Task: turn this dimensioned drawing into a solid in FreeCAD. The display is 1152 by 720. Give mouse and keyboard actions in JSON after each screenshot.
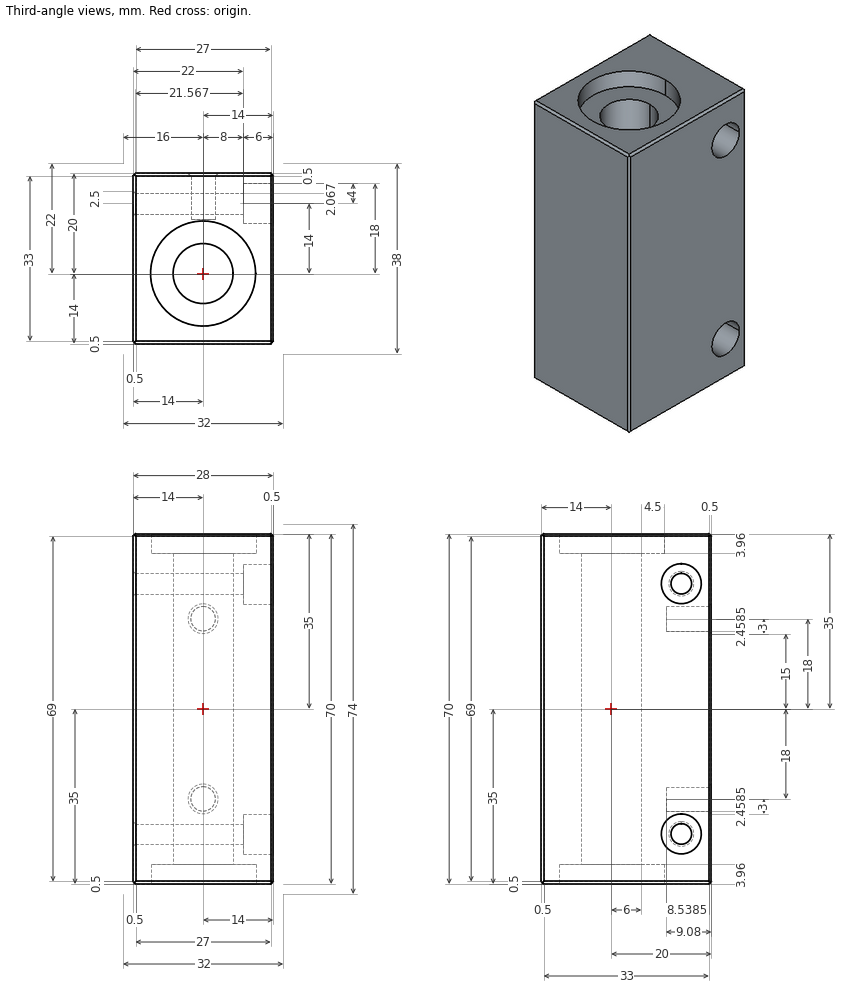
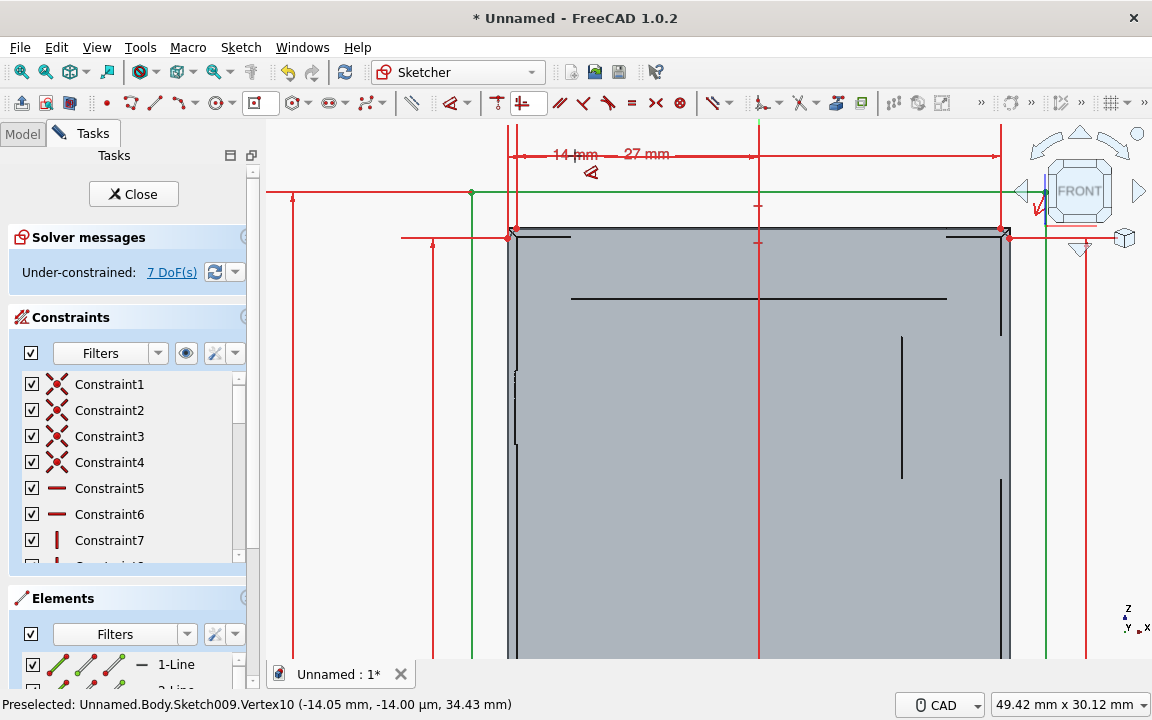
{"action": "scroll", "coordinate": [602, 236], "scroll_direction": "down", "scroll_amount": 7}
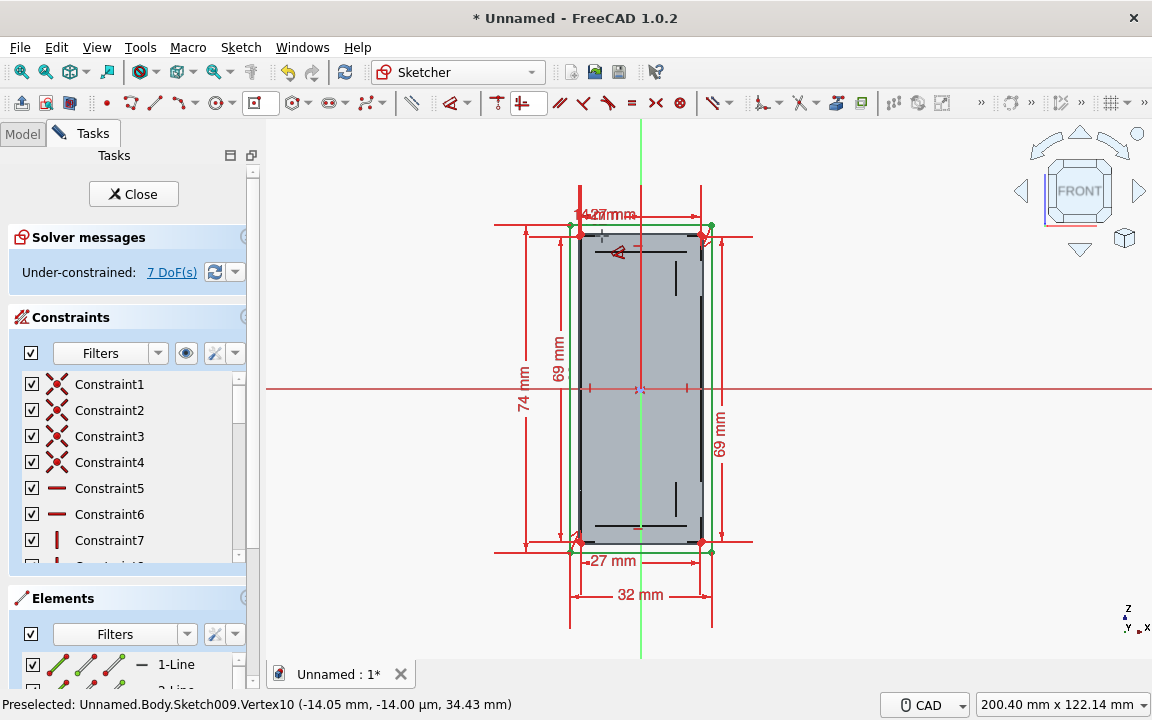
{"action": "scroll", "coordinate": [581, 544], "scroll_direction": "up", "scroll_amount": 8}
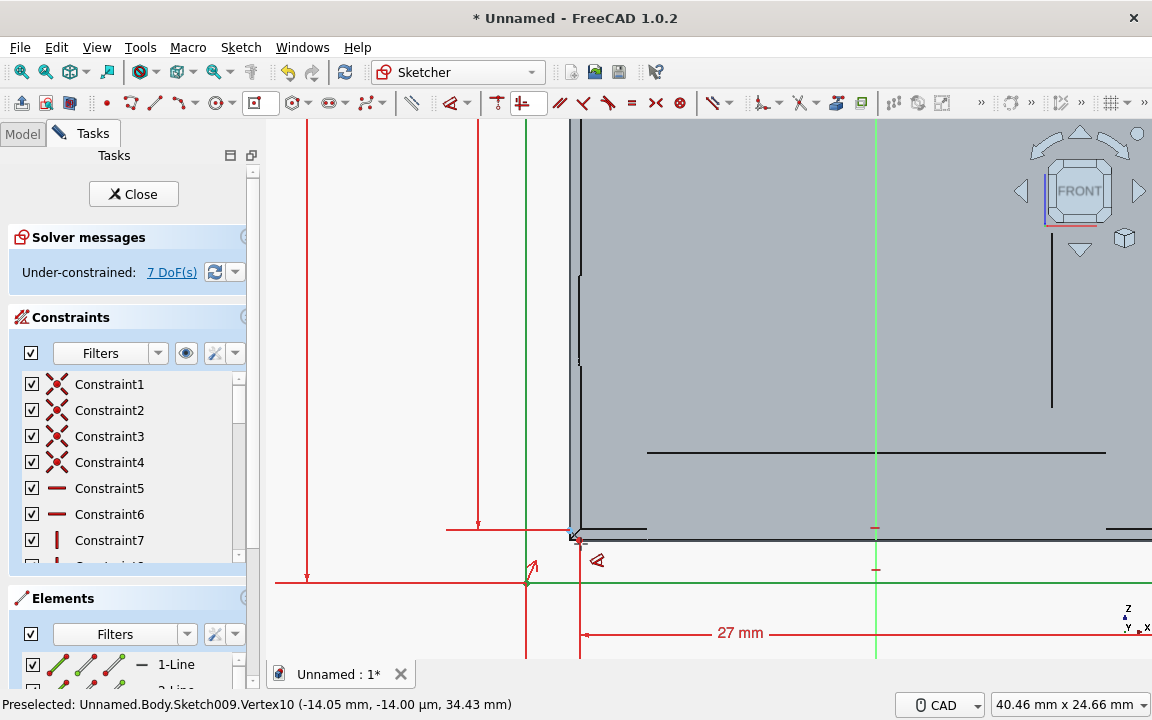
{"action": "left_click", "coordinate": [580, 541]}
{"action": "left_click", "coordinate": [546, 344]}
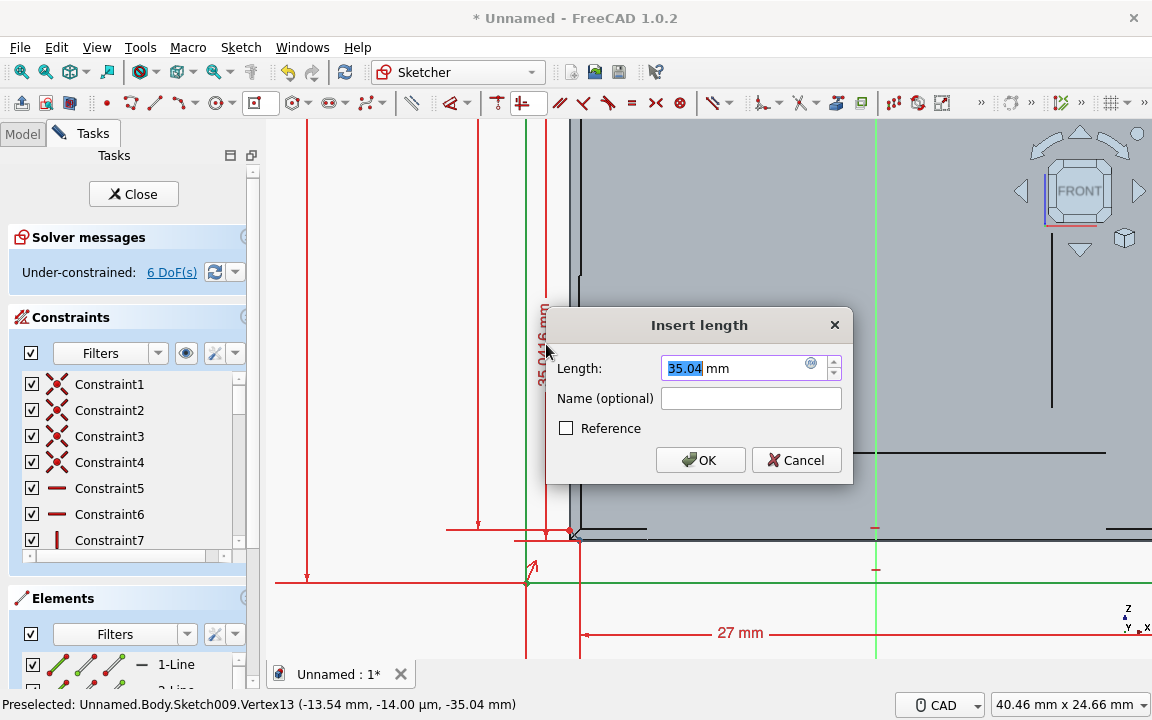
{"action": "type", "text": "35"}
{"action": "key", "text": "Return"}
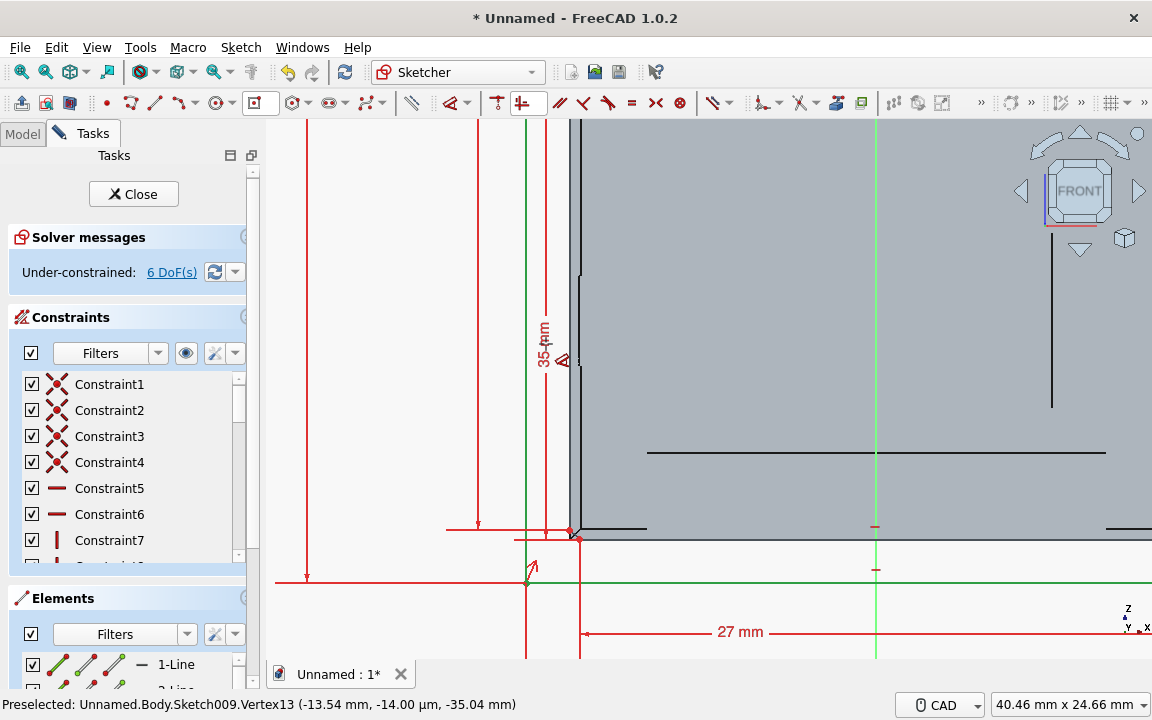
{"action": "scroll", "coordinate": [581, 545], "scroll_direction": "down", "scroll_amount": 8}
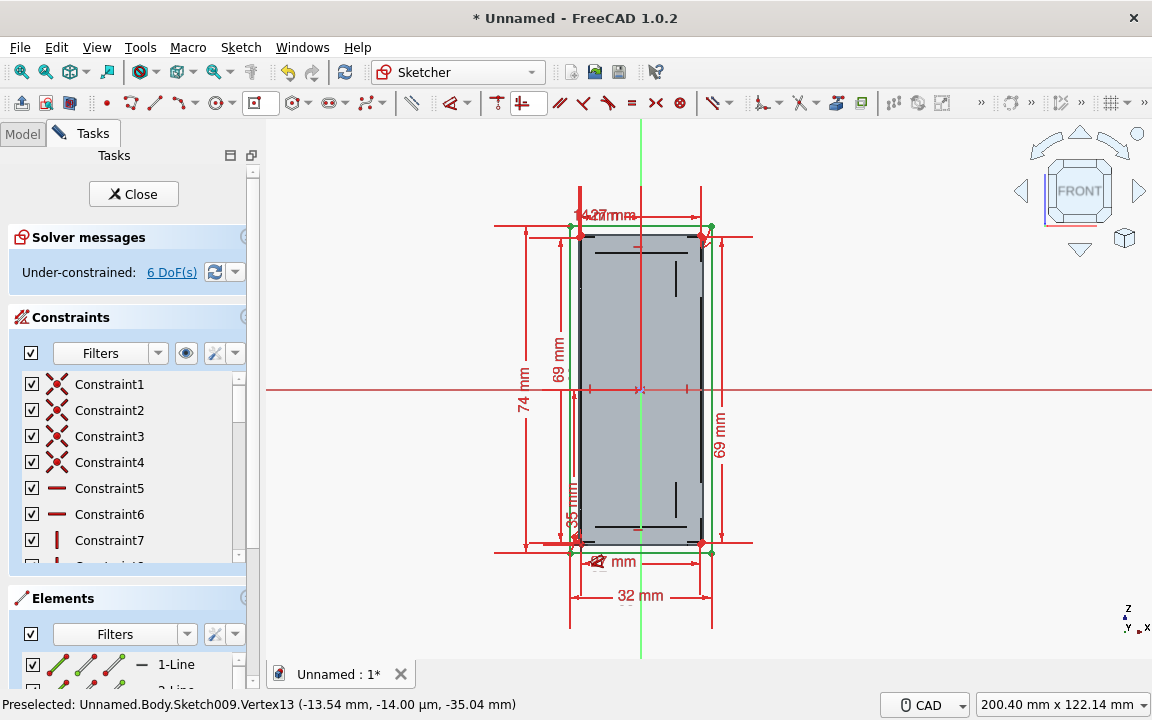
{"action": "scroll", "coordinate": [703, 543], "scroll_direction": "up", "scroll_amount": 7}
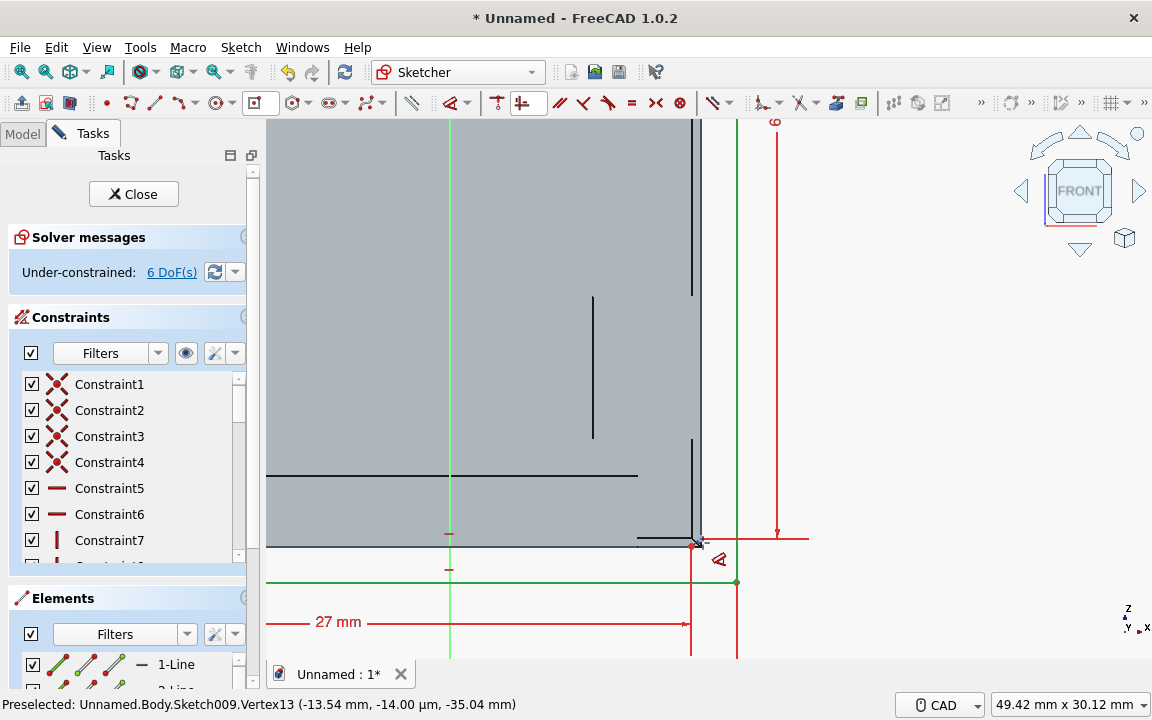
{"action": "left_click", "coordinate": [701, 539]}
{"action": "left_click", "coordinate": [575, 597]}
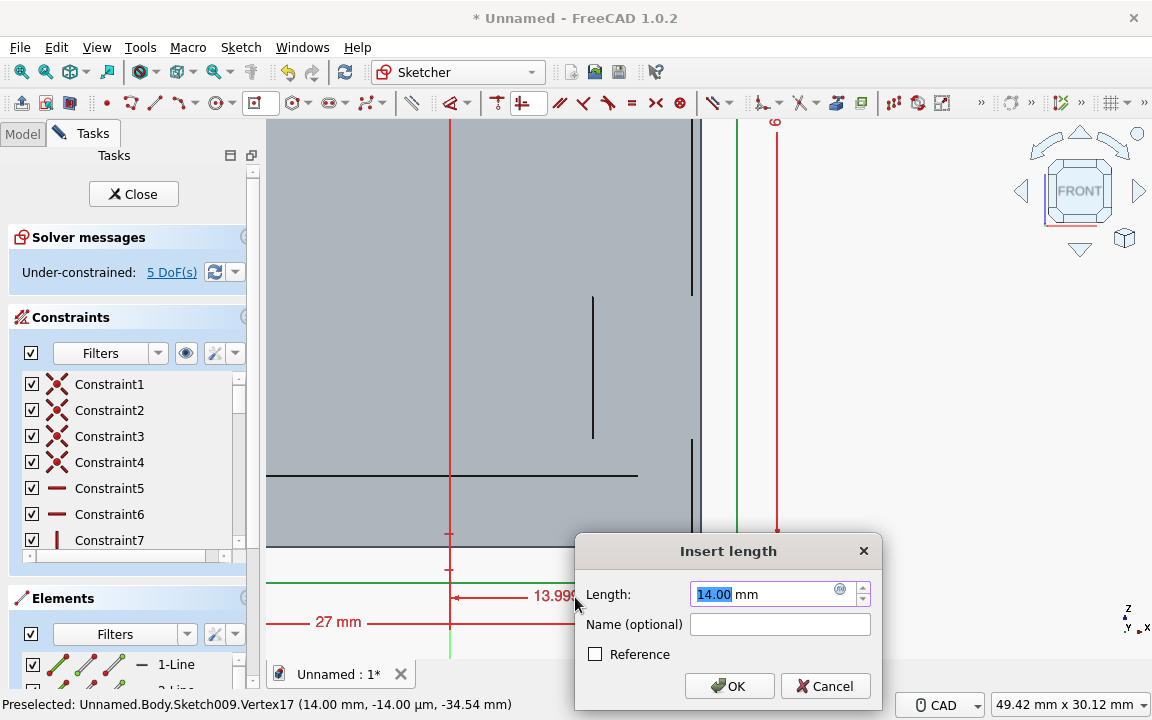
{"action": "type", "text": "14"}
{"action": "key", "text": "Return"}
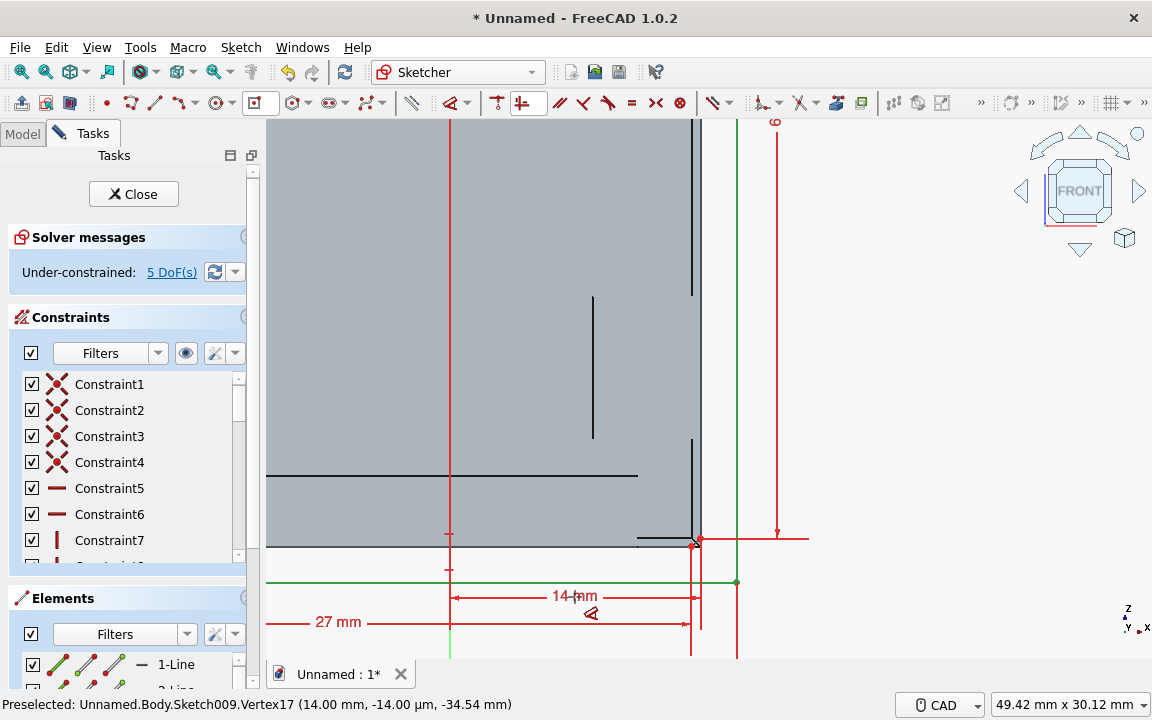
{"action": "scroll", "coordinate": [703, 543], "scroll_direction": "down", "scroll_amount": 7}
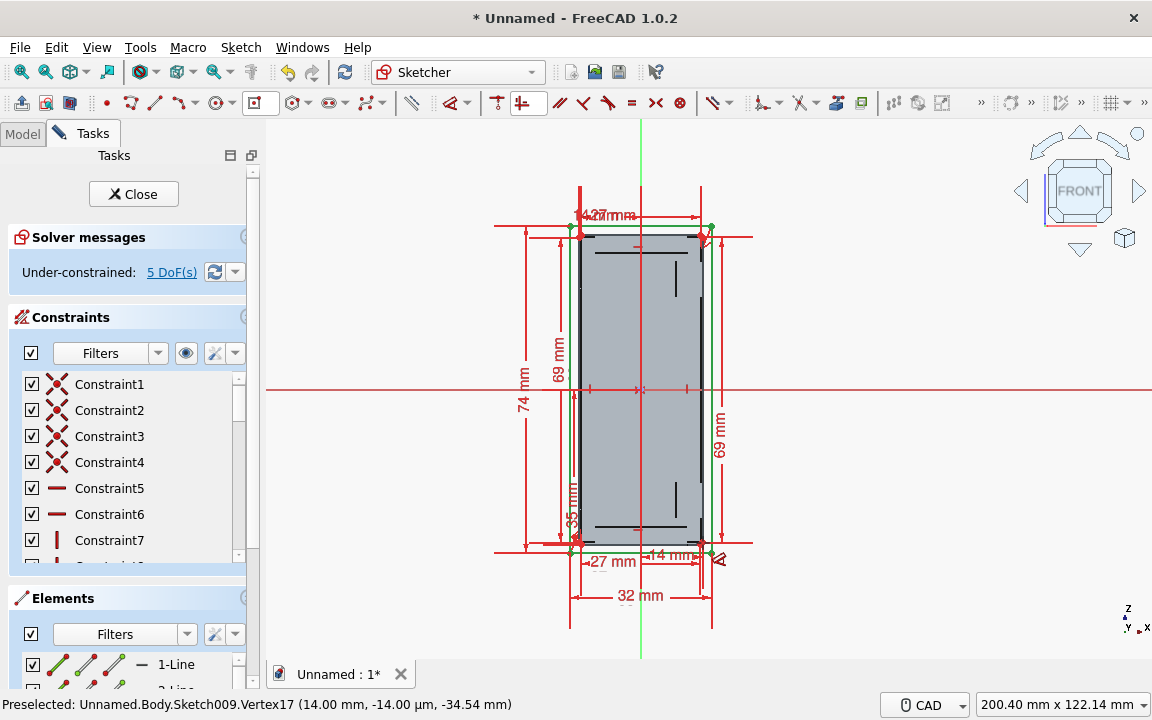
{"action": "scroll", "coordinate": [701, 235], "scroll_direction": "up", "scroll_amount": 7}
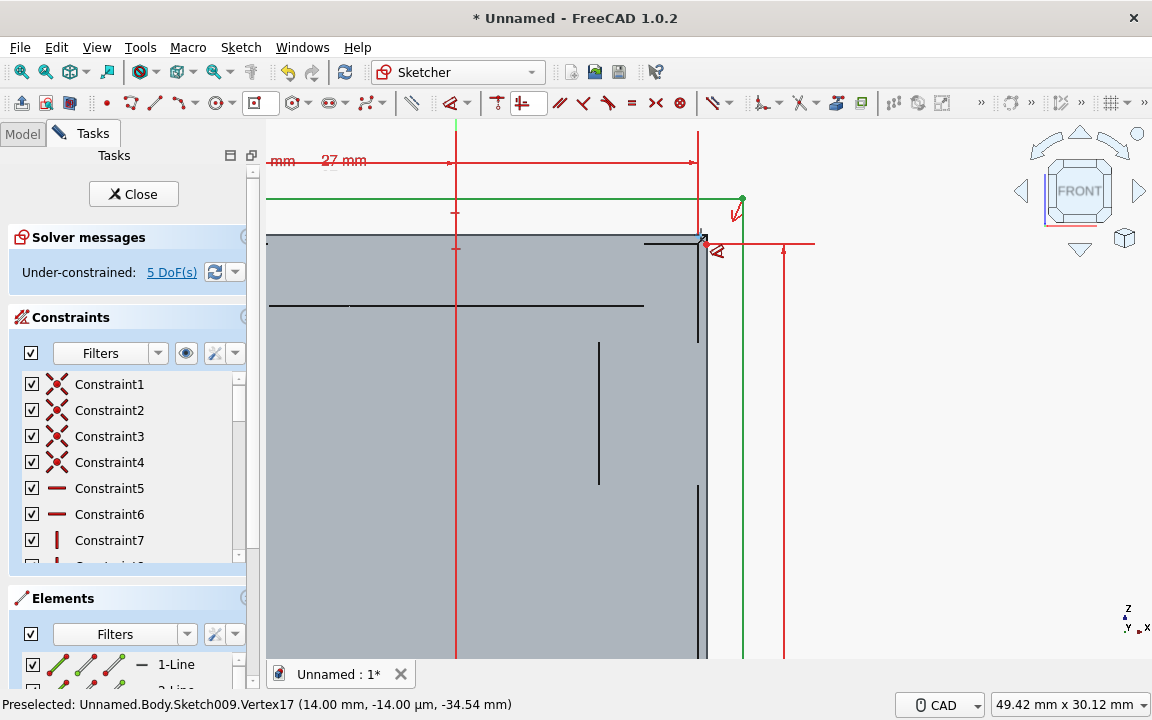
{"action": "left_click", "coordinate": [698, 235]}
{"action": "left_click", "coordinate": [422, 433]}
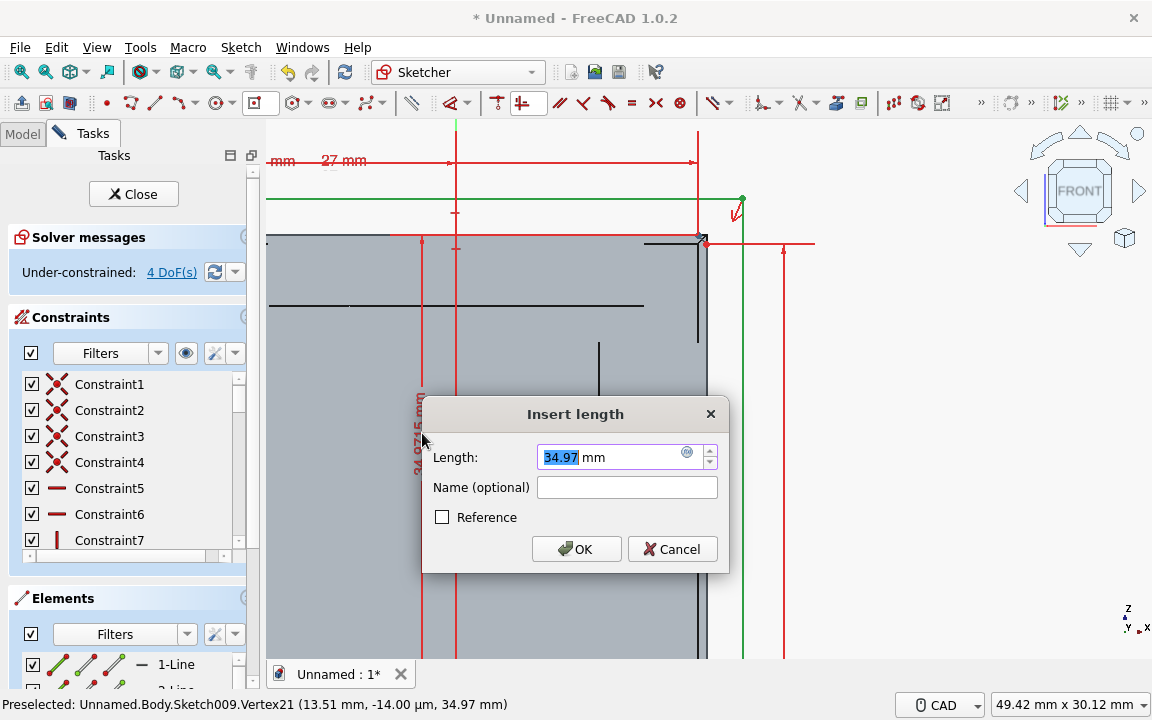
{"action": "type", "text": "35"}
{"action": "key", "text": "Return"}